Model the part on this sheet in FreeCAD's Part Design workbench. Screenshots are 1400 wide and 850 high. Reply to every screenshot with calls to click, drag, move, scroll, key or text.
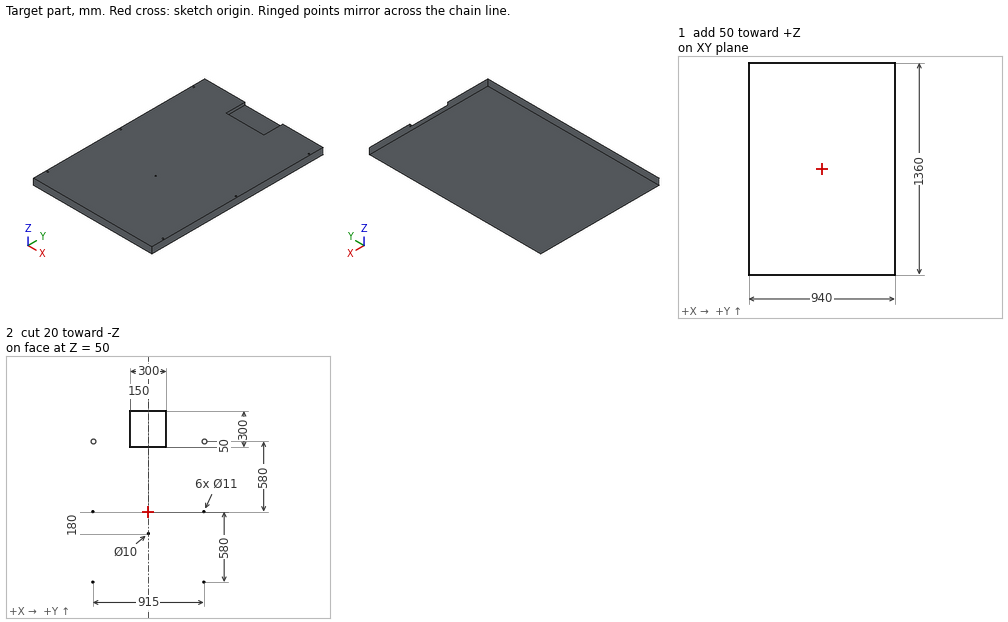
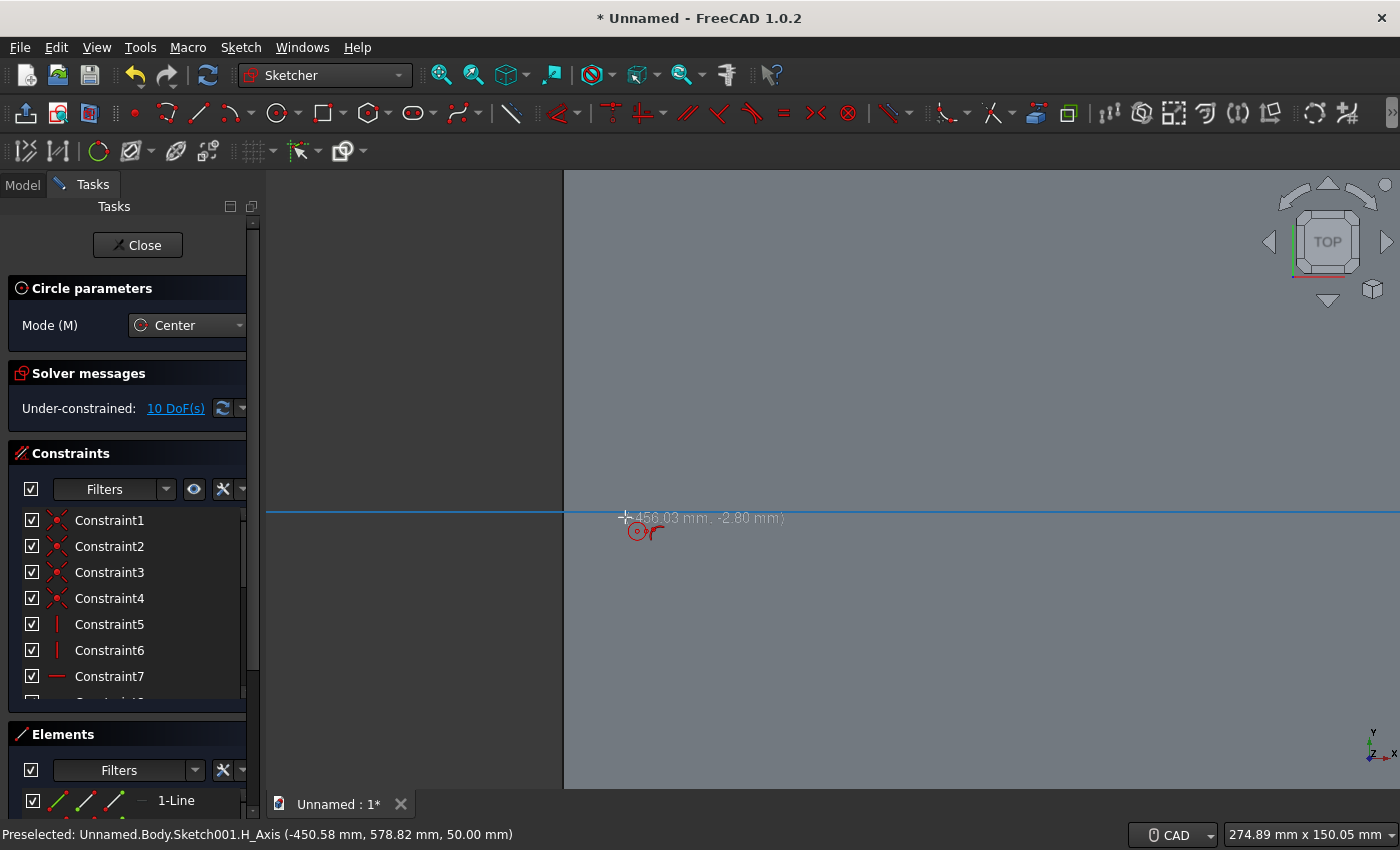
scroll(625, 517, down, 13)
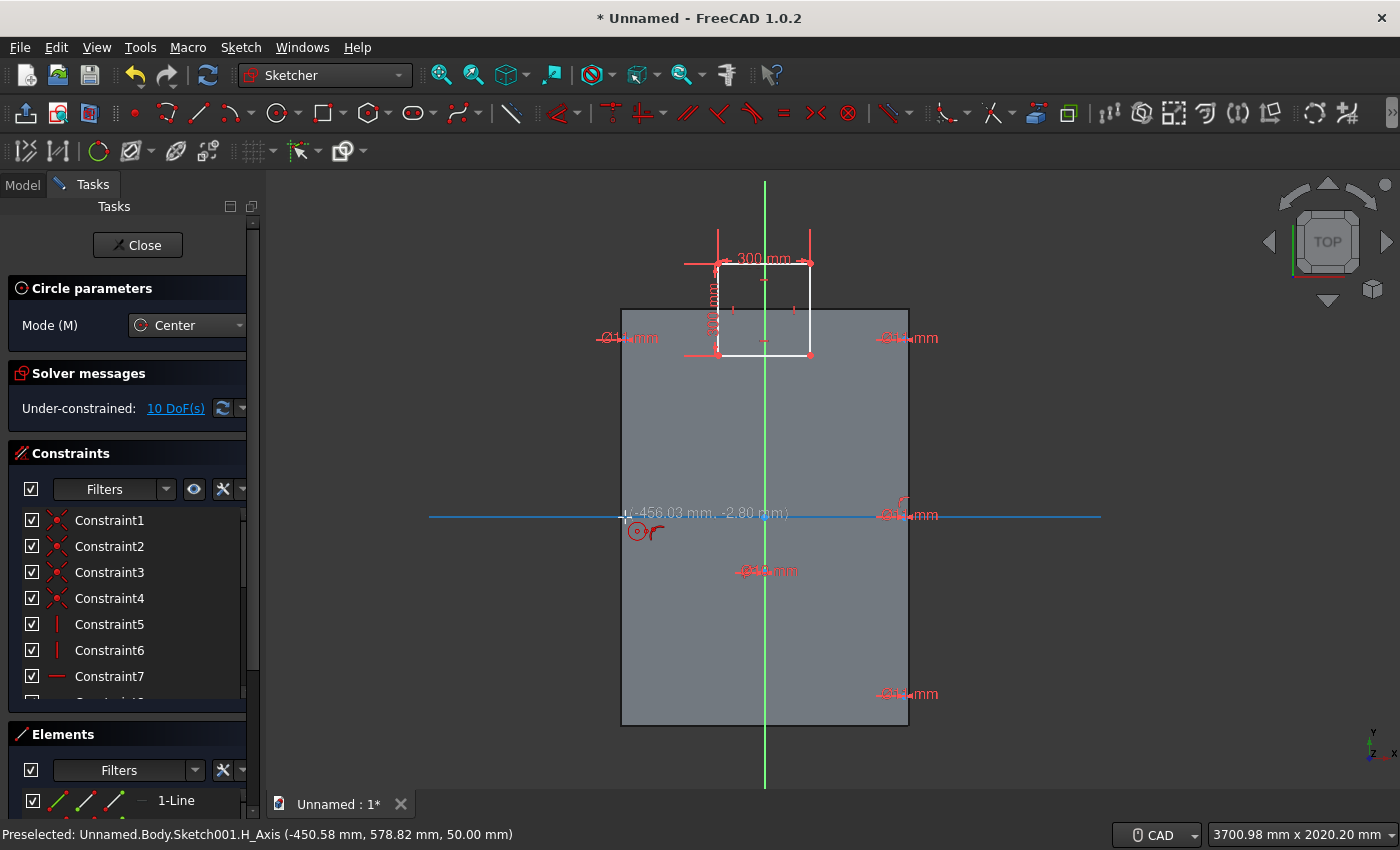
click(625, 517)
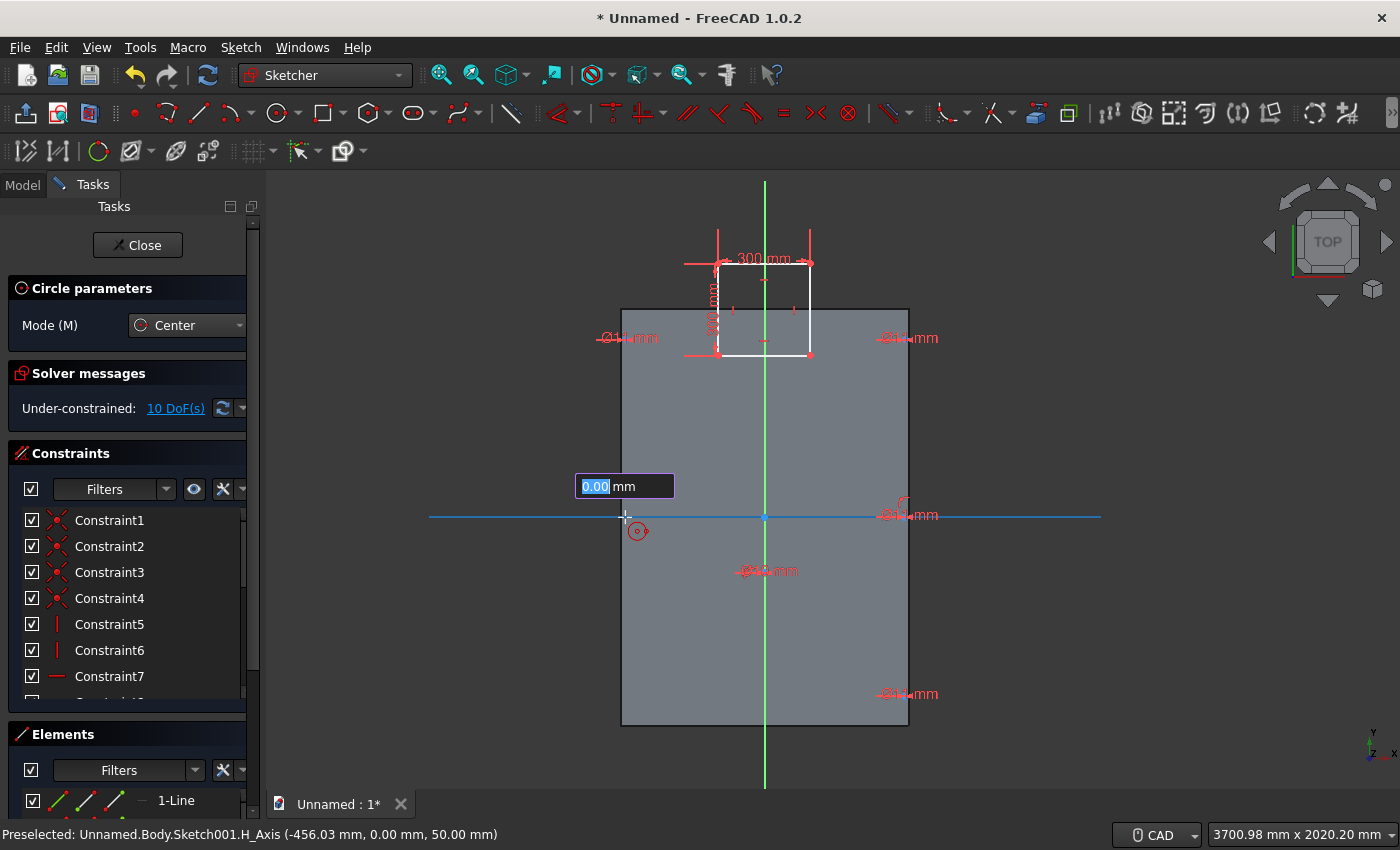
scroll(625, 516, up, 12)
move(623, 506)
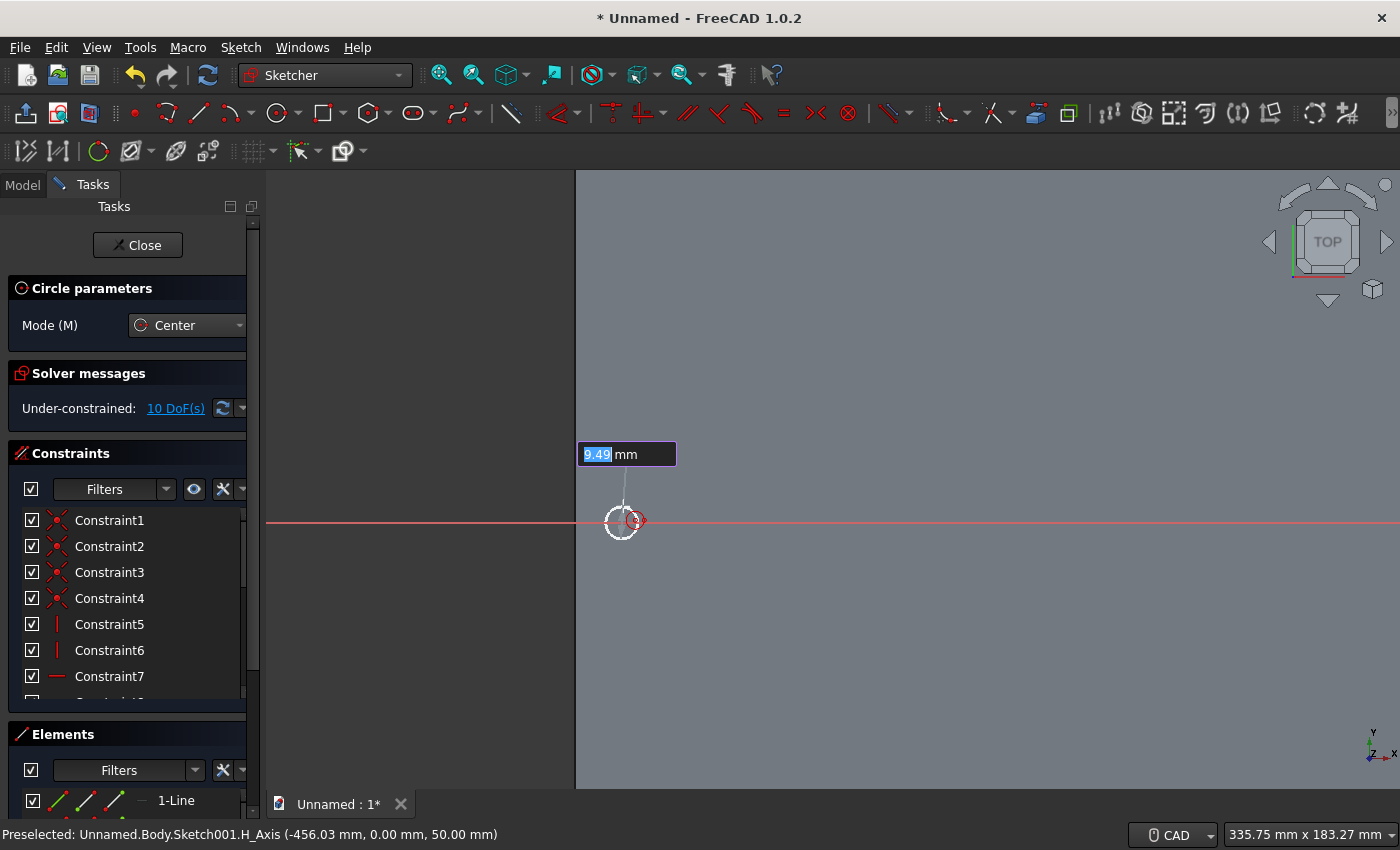
text(11)
key(Return)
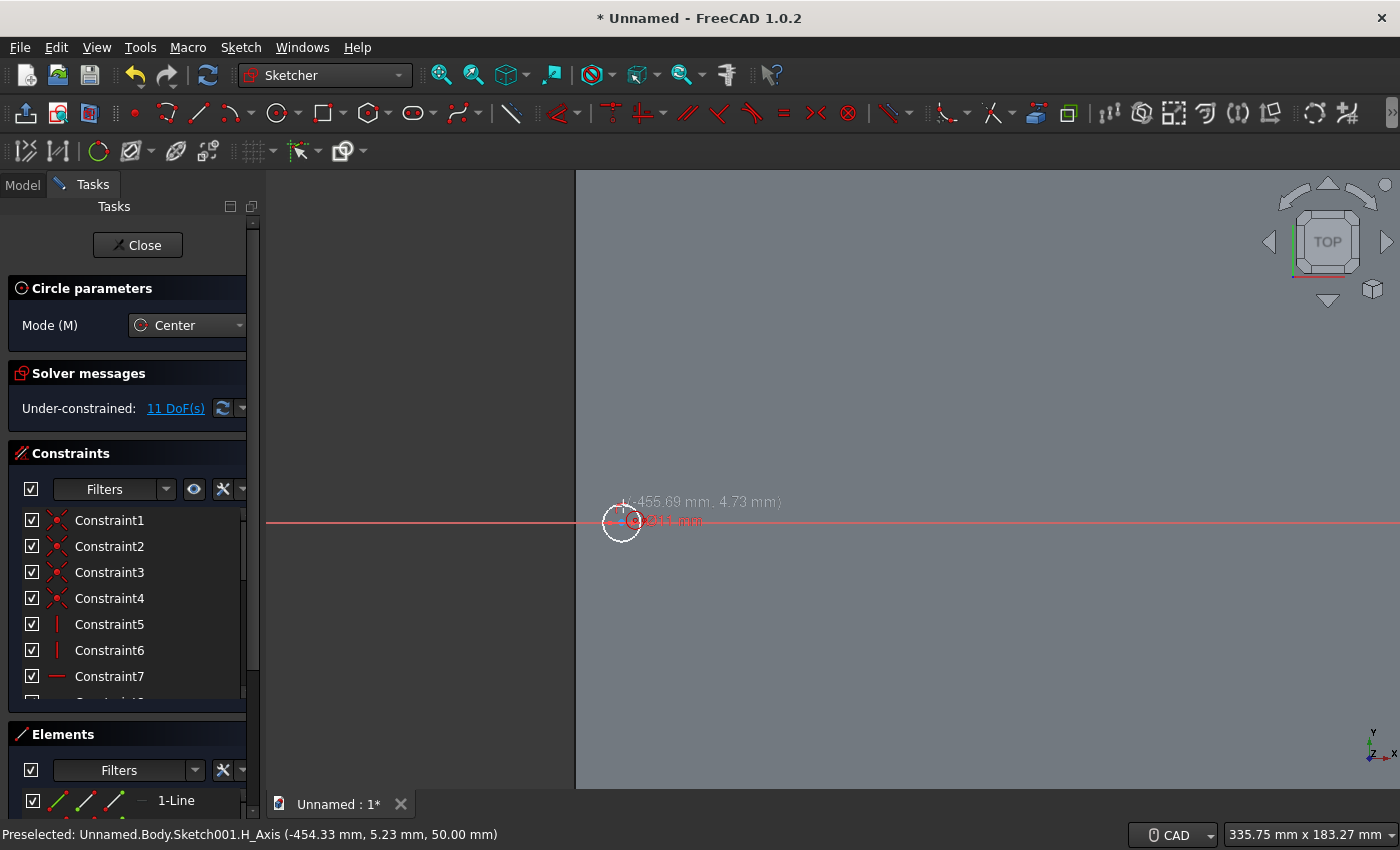
scroll(625, 516, down, 12)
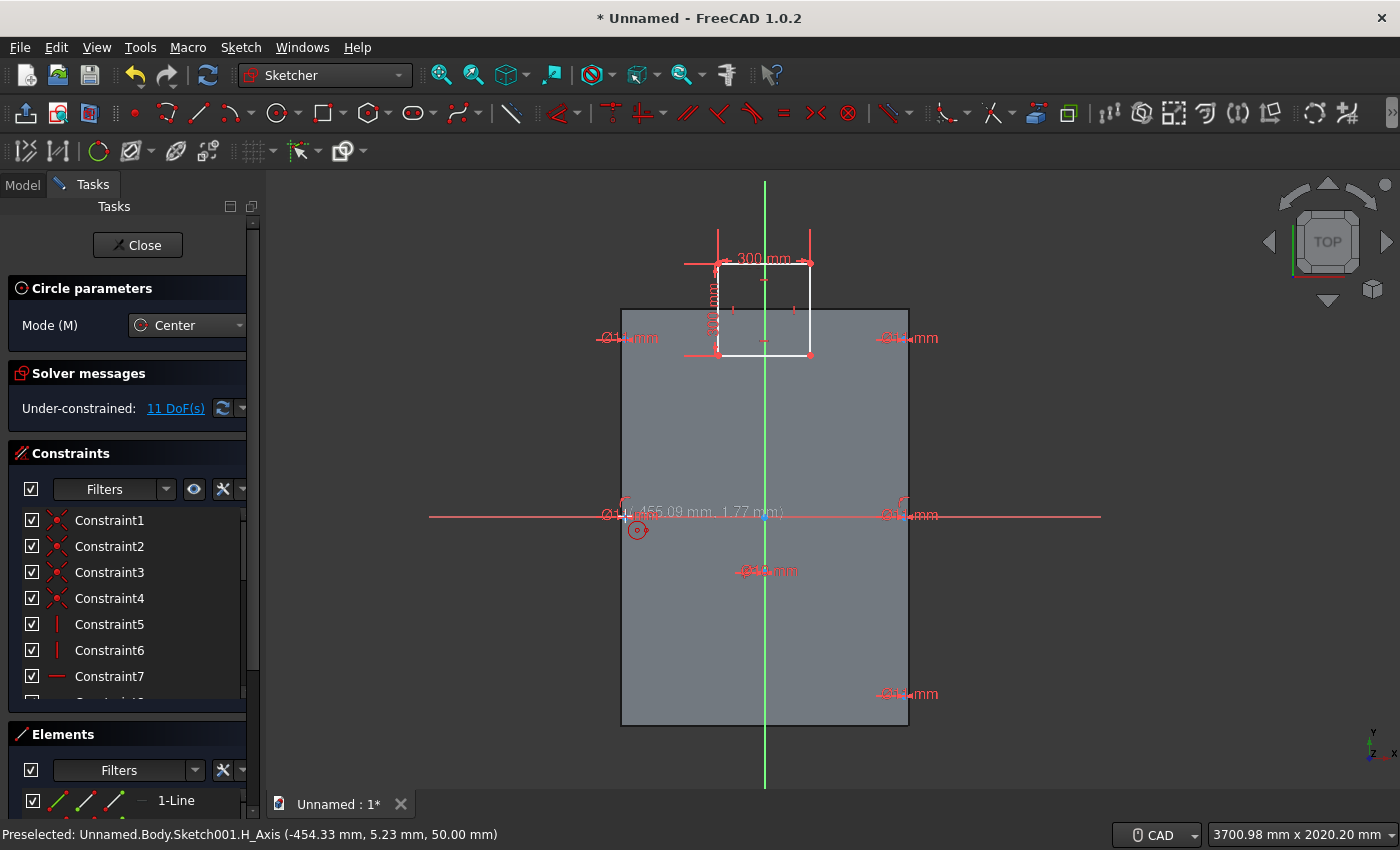
scroll(625, 695, up, 13)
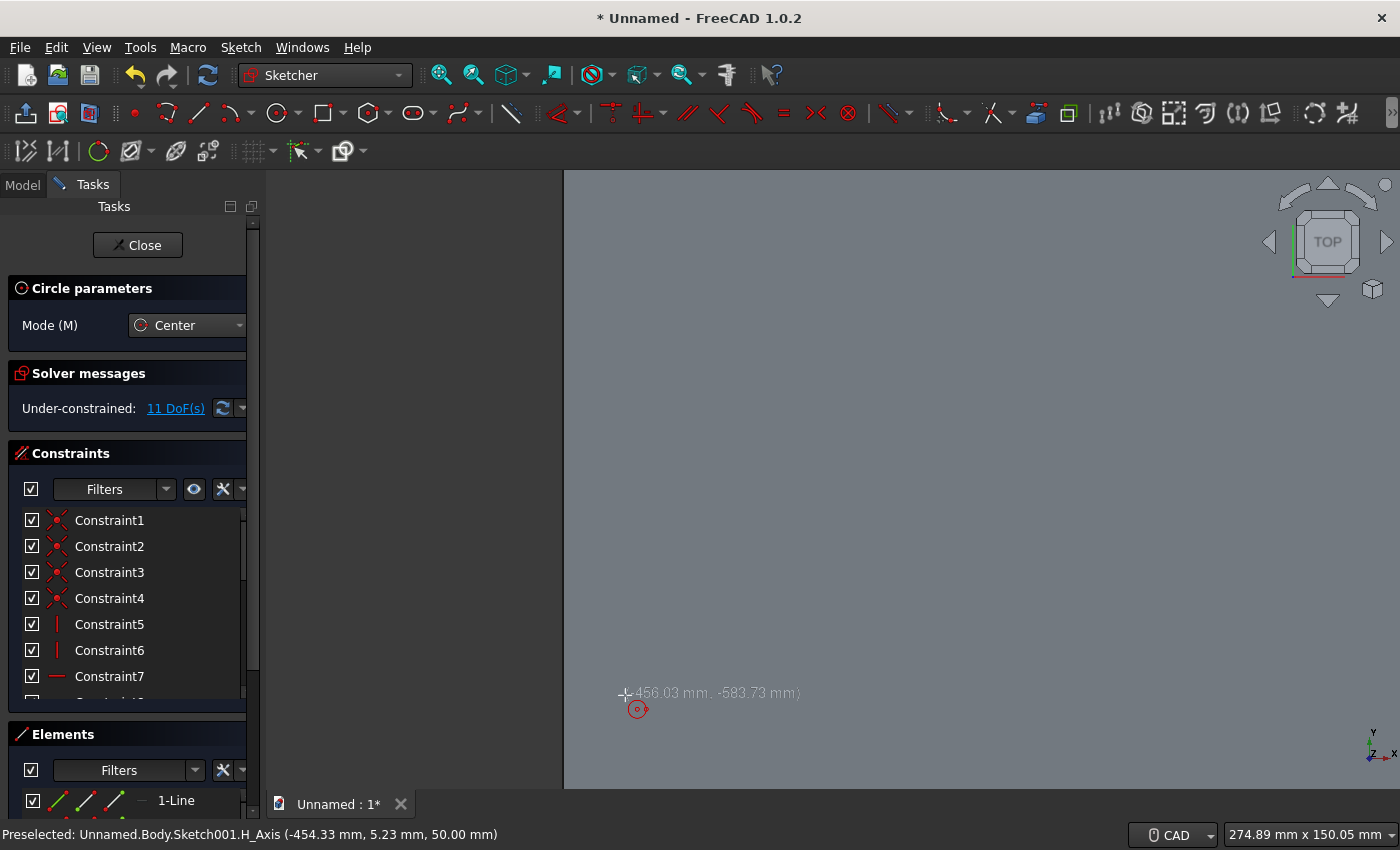
scroll(625, 696, down, 13)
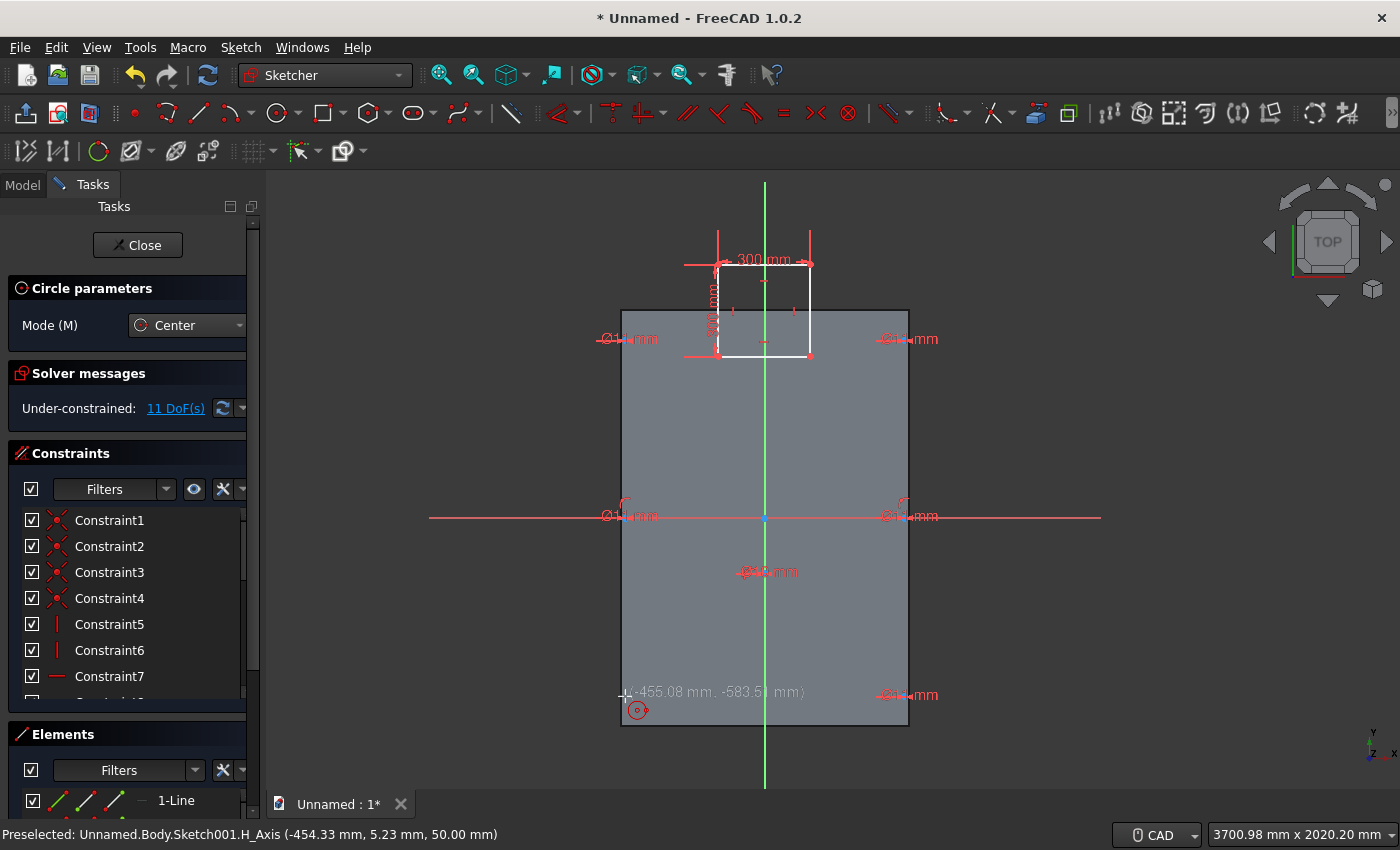
click(625, 696)
move(626, 695)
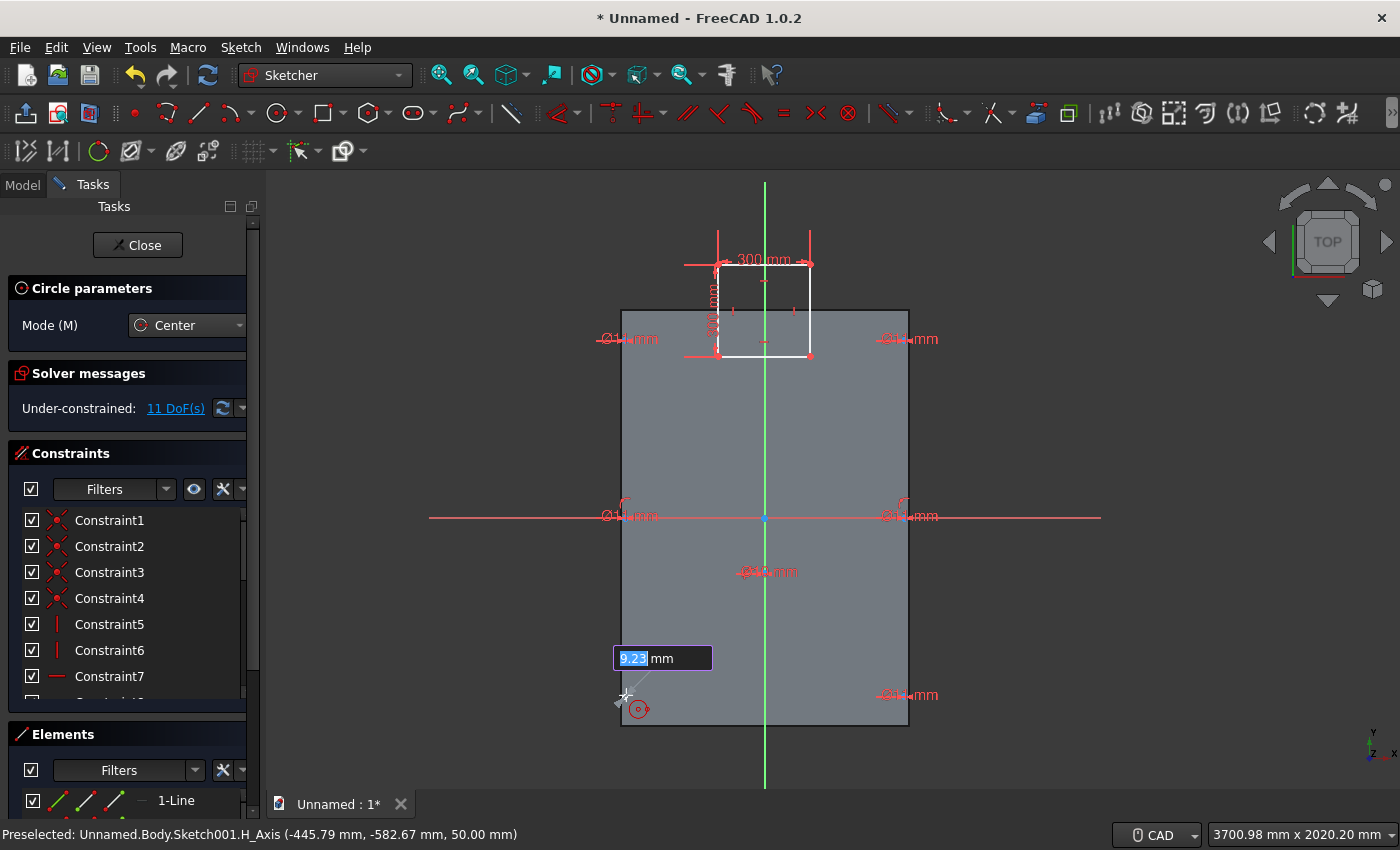
text(11)
key(Return)
key(Escape)